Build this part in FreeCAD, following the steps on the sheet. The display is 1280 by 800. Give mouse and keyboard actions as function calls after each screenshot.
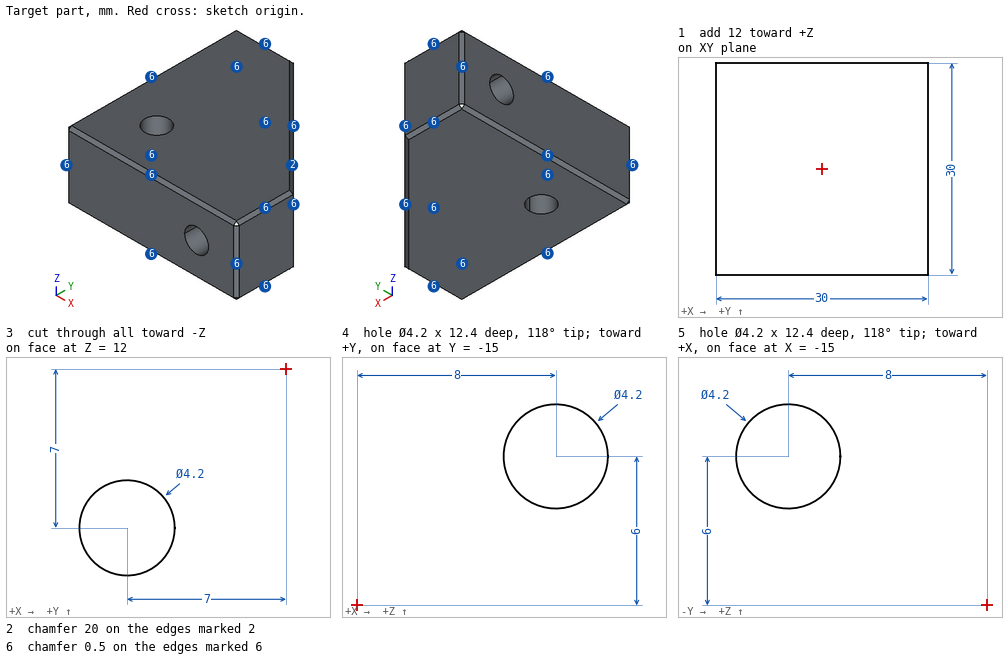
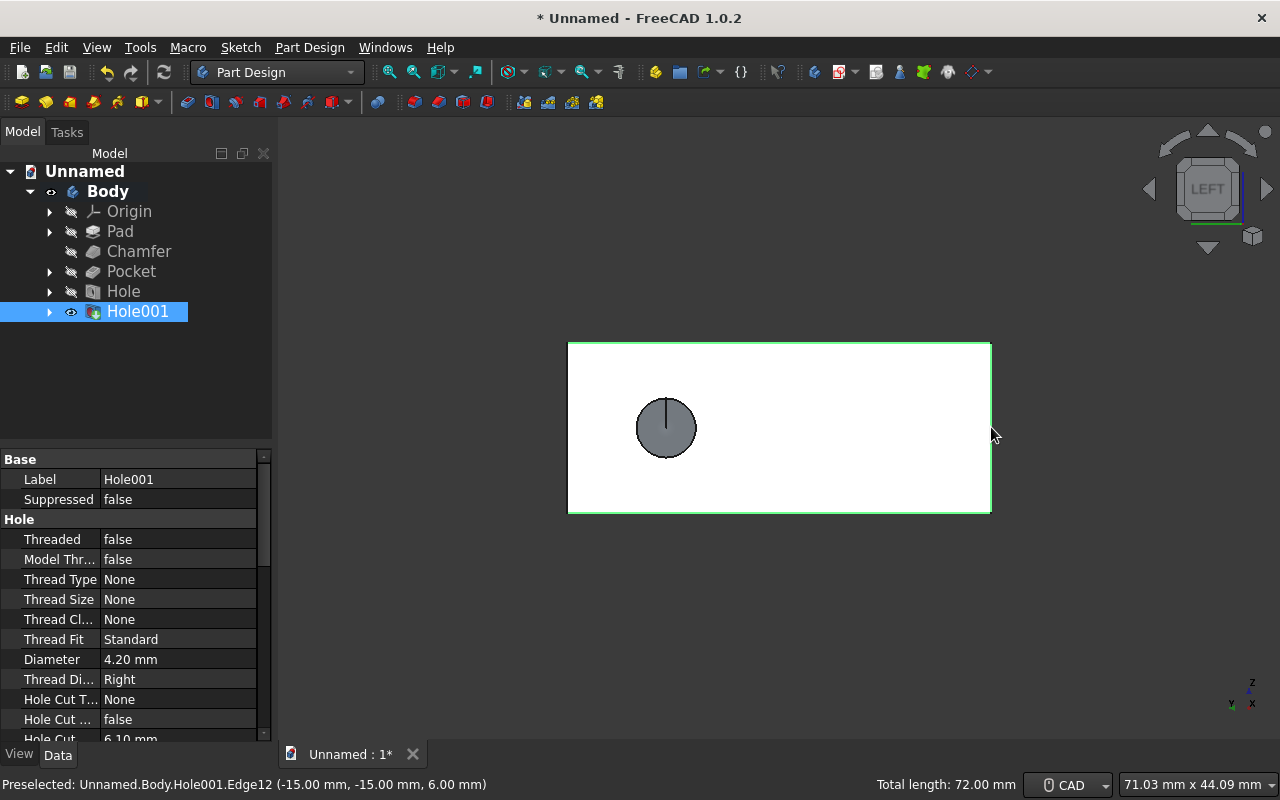
click(567, 427, ctrl)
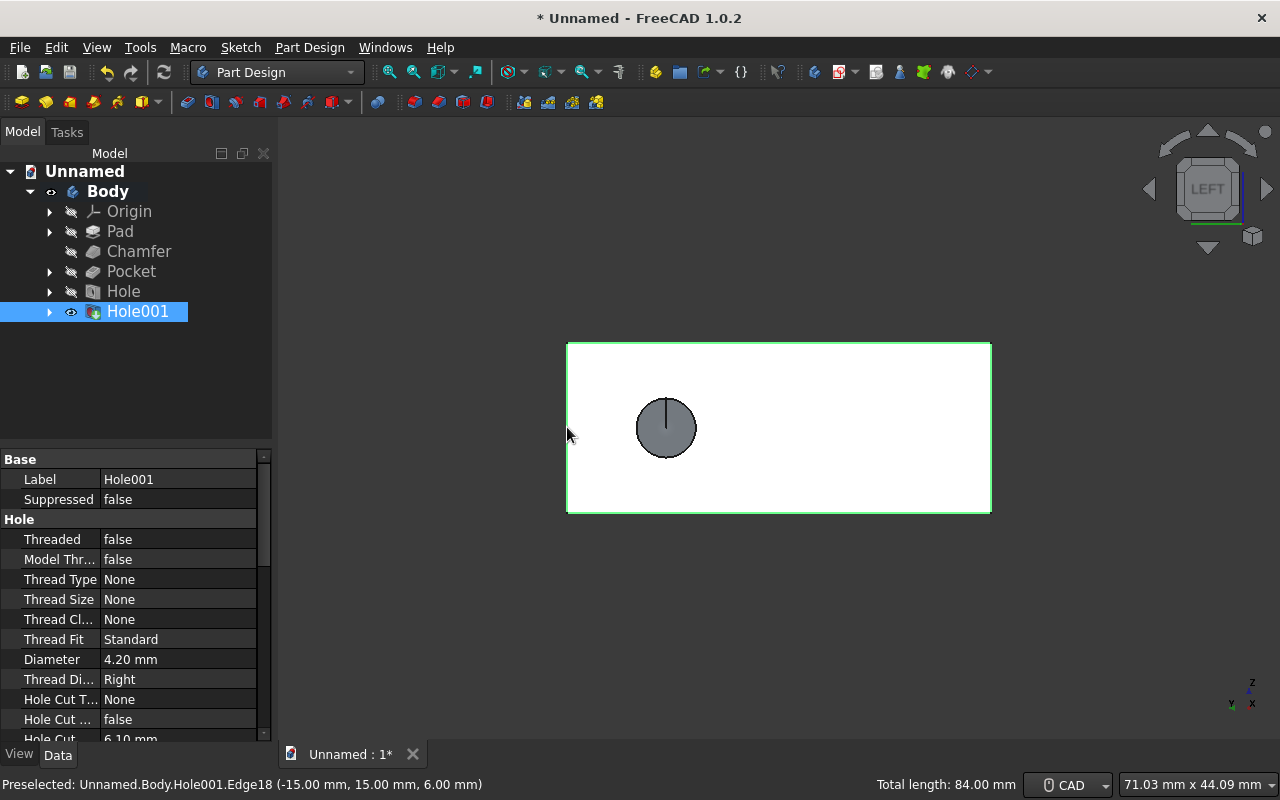
key(0)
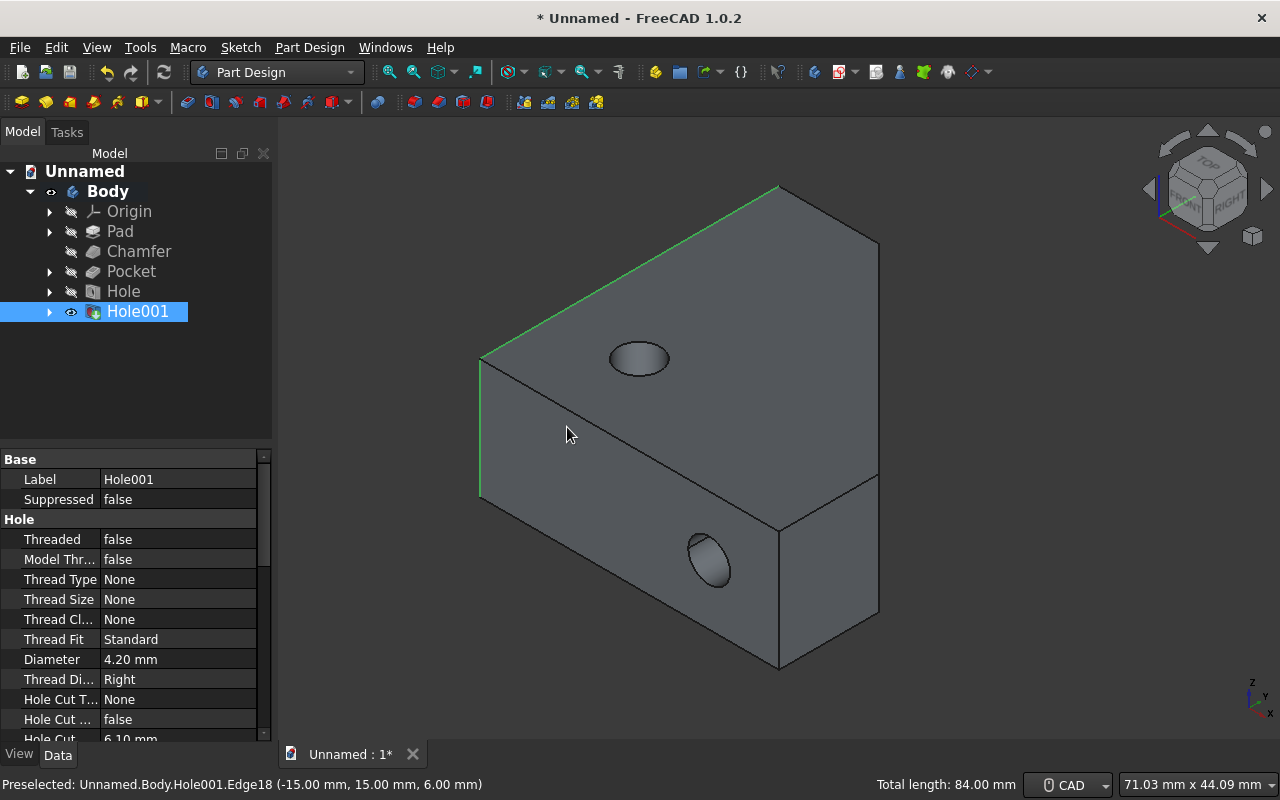
click(879, 358, ctrl)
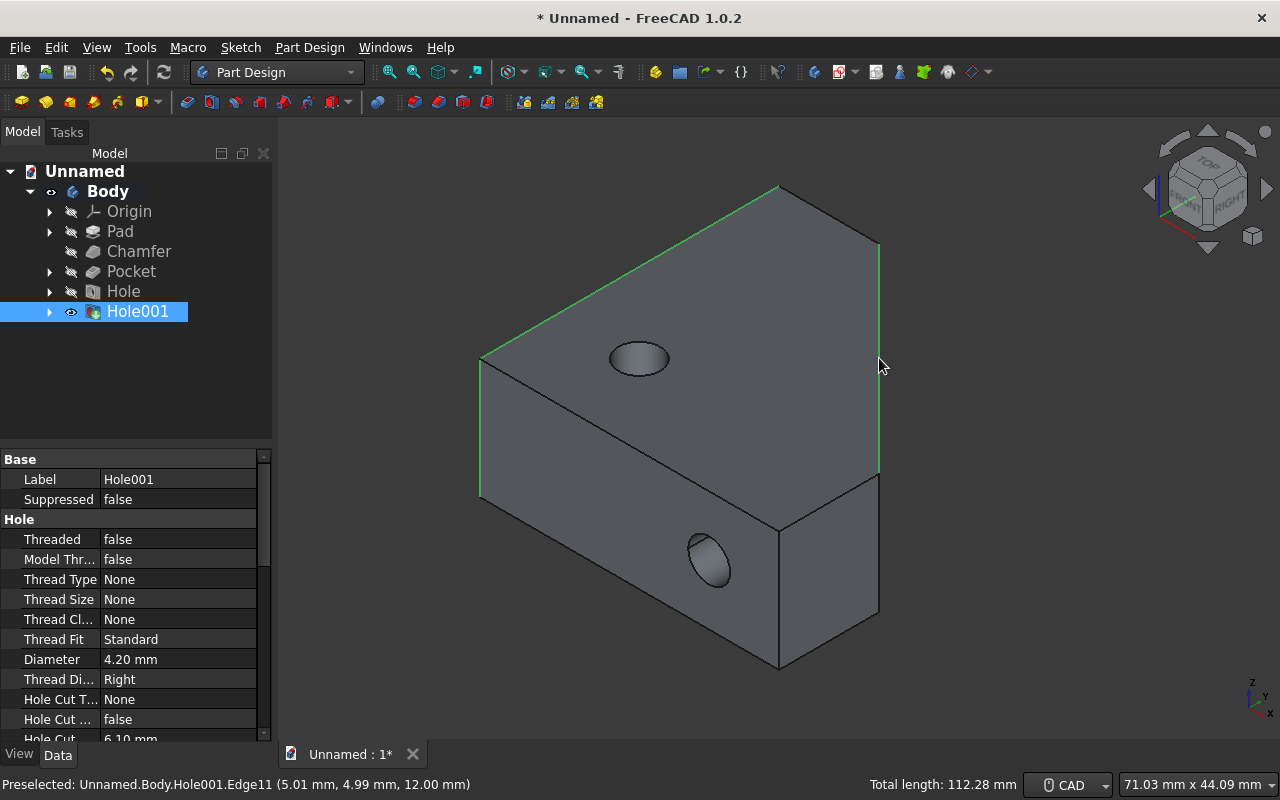
click(629, 444, ctrl)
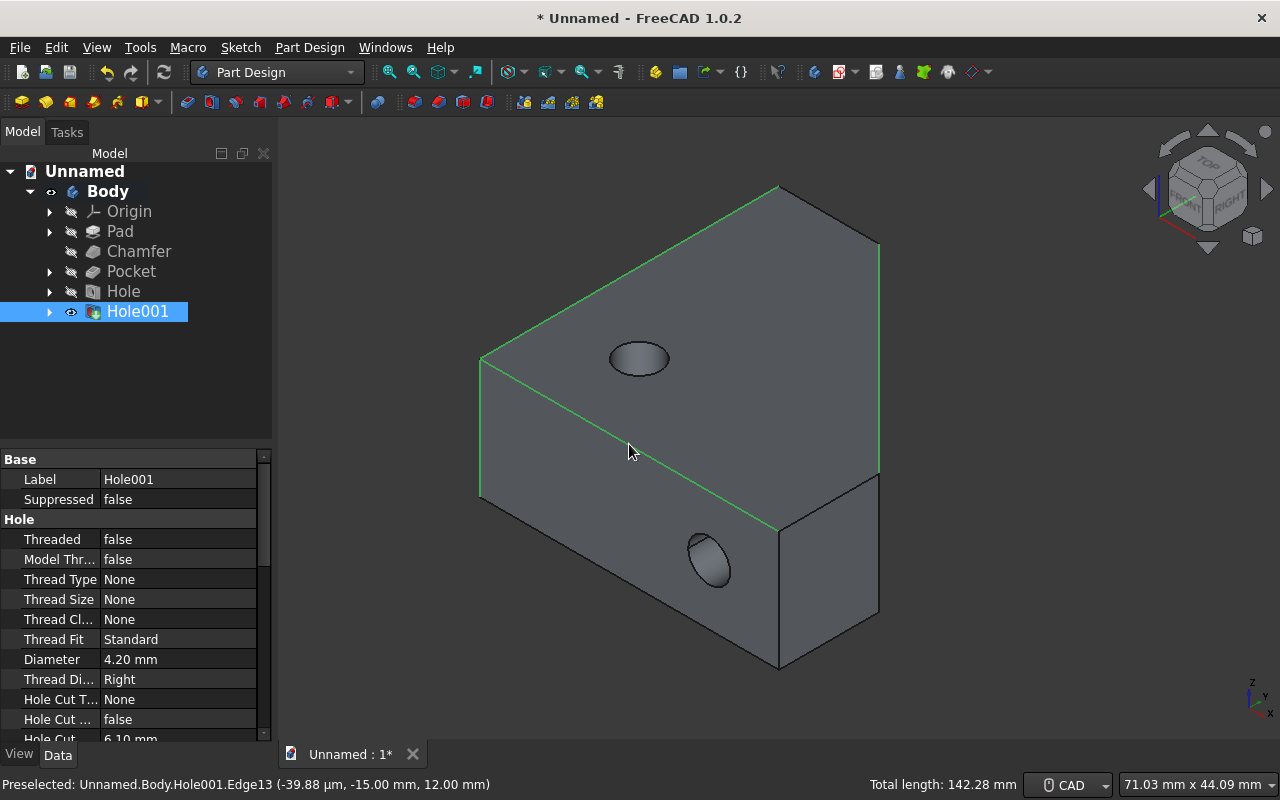
click(829, 502, ctrl)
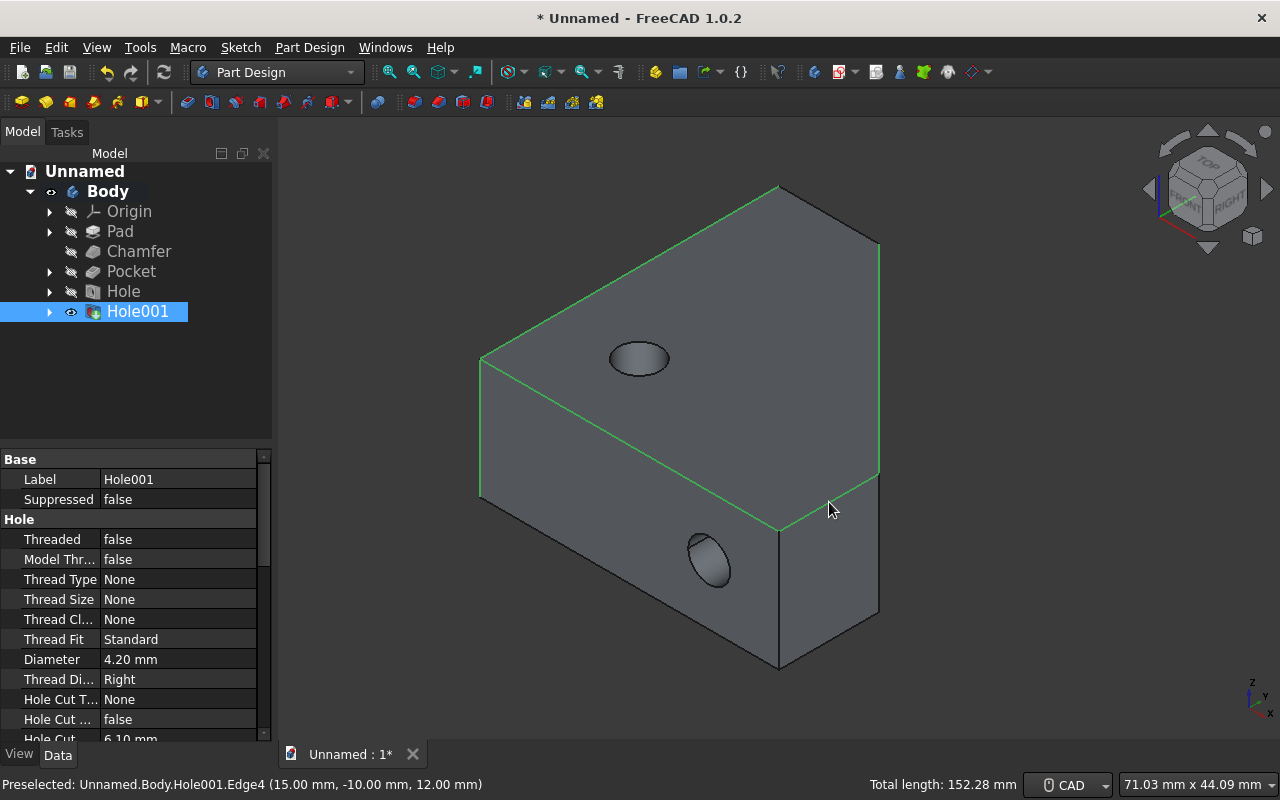
click(779, 600, ctrl)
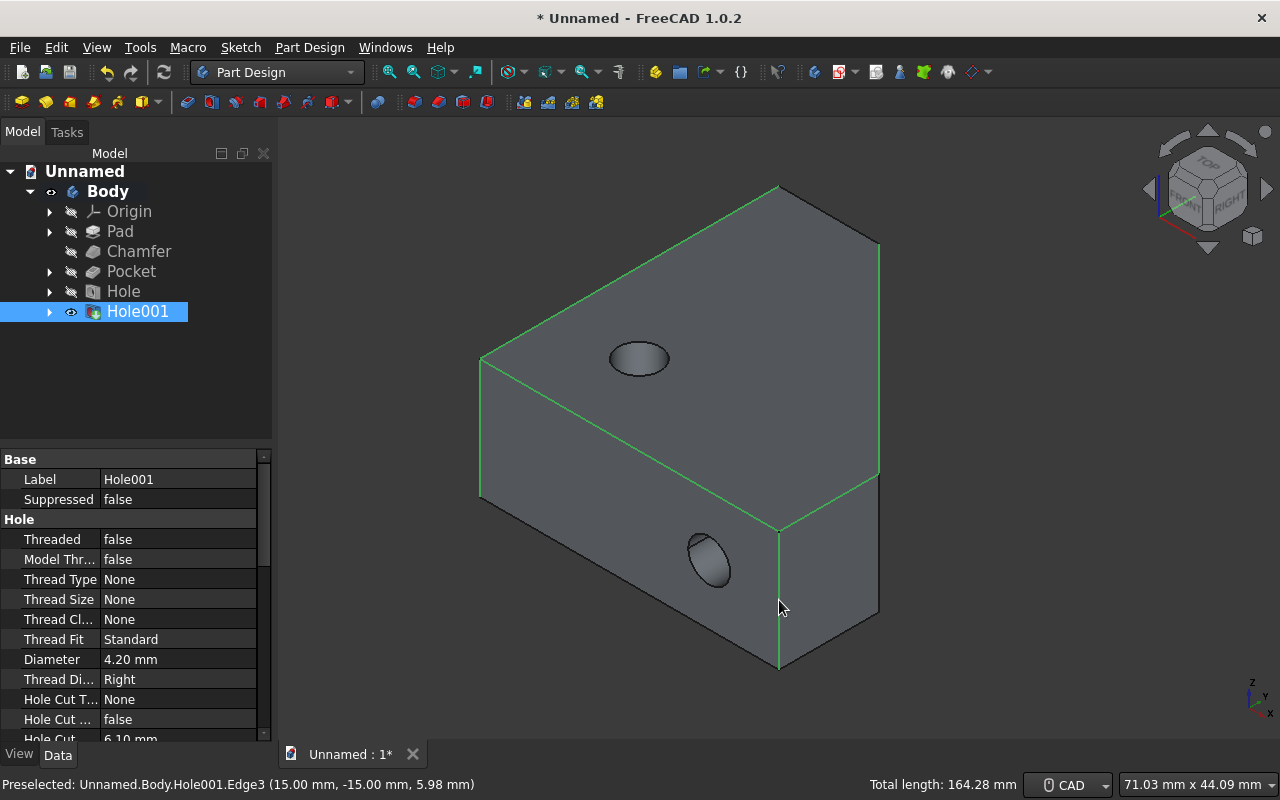
key(2)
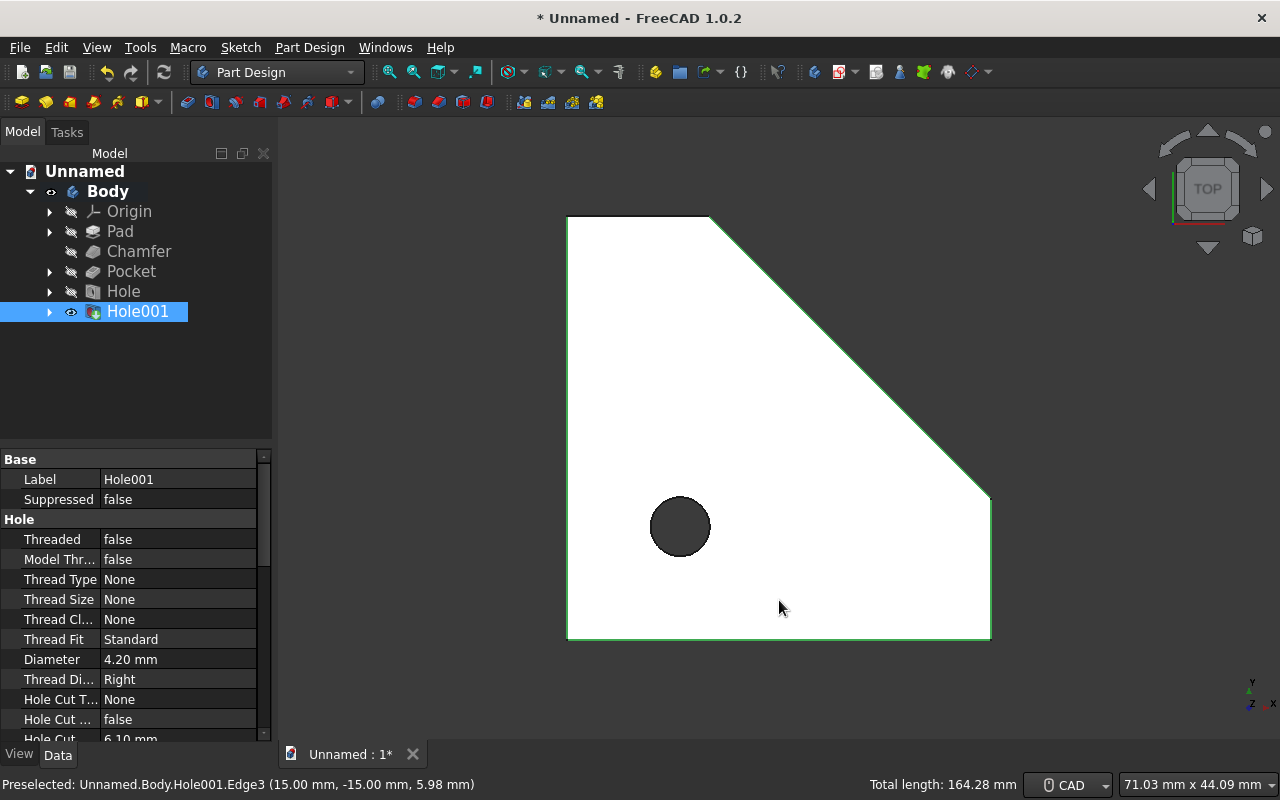
click(638, 215, ctrl)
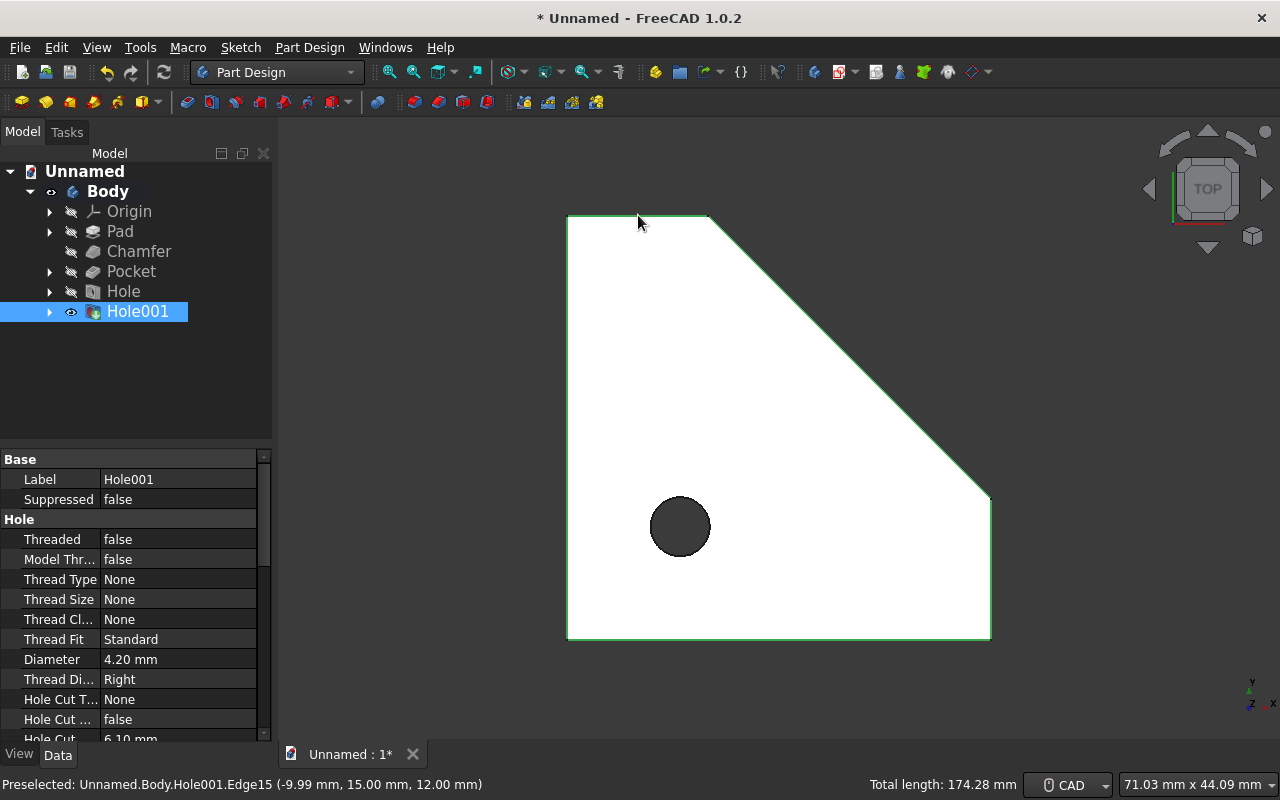
key(1)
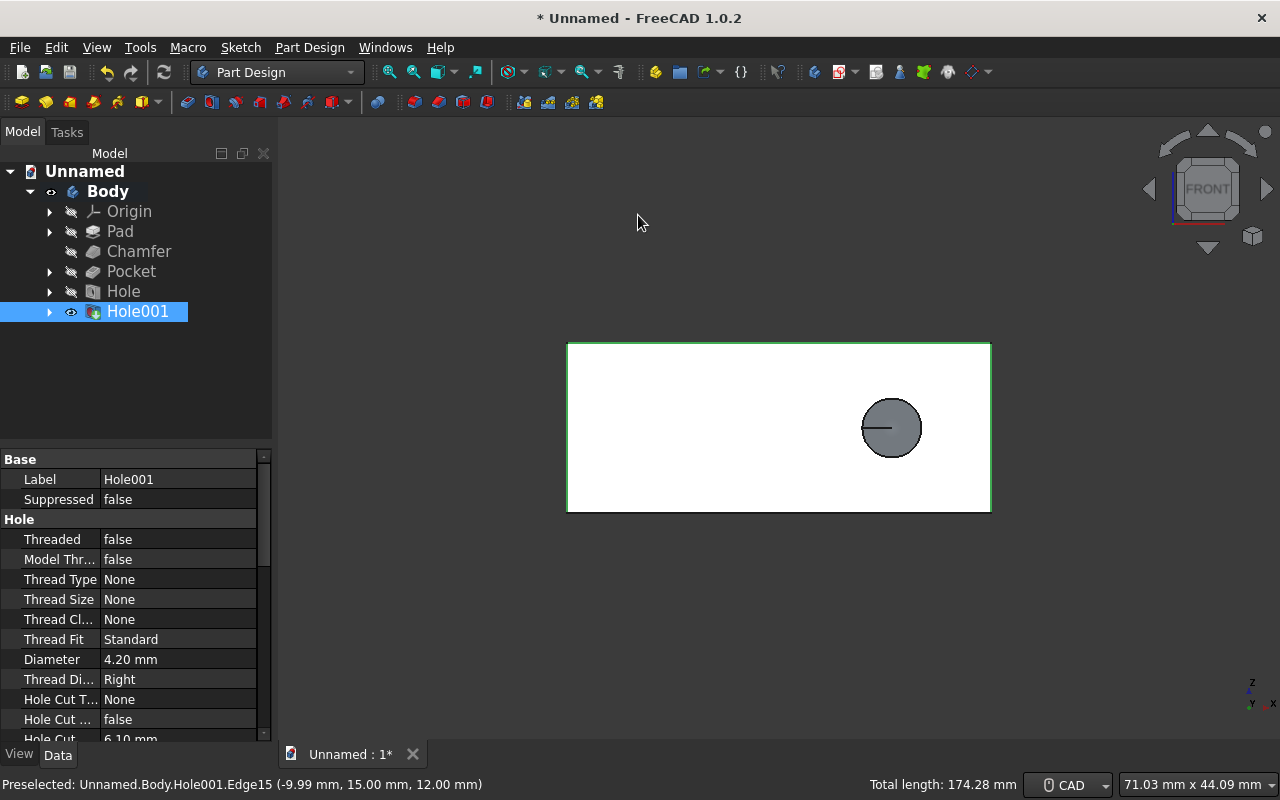
click(390, 72)